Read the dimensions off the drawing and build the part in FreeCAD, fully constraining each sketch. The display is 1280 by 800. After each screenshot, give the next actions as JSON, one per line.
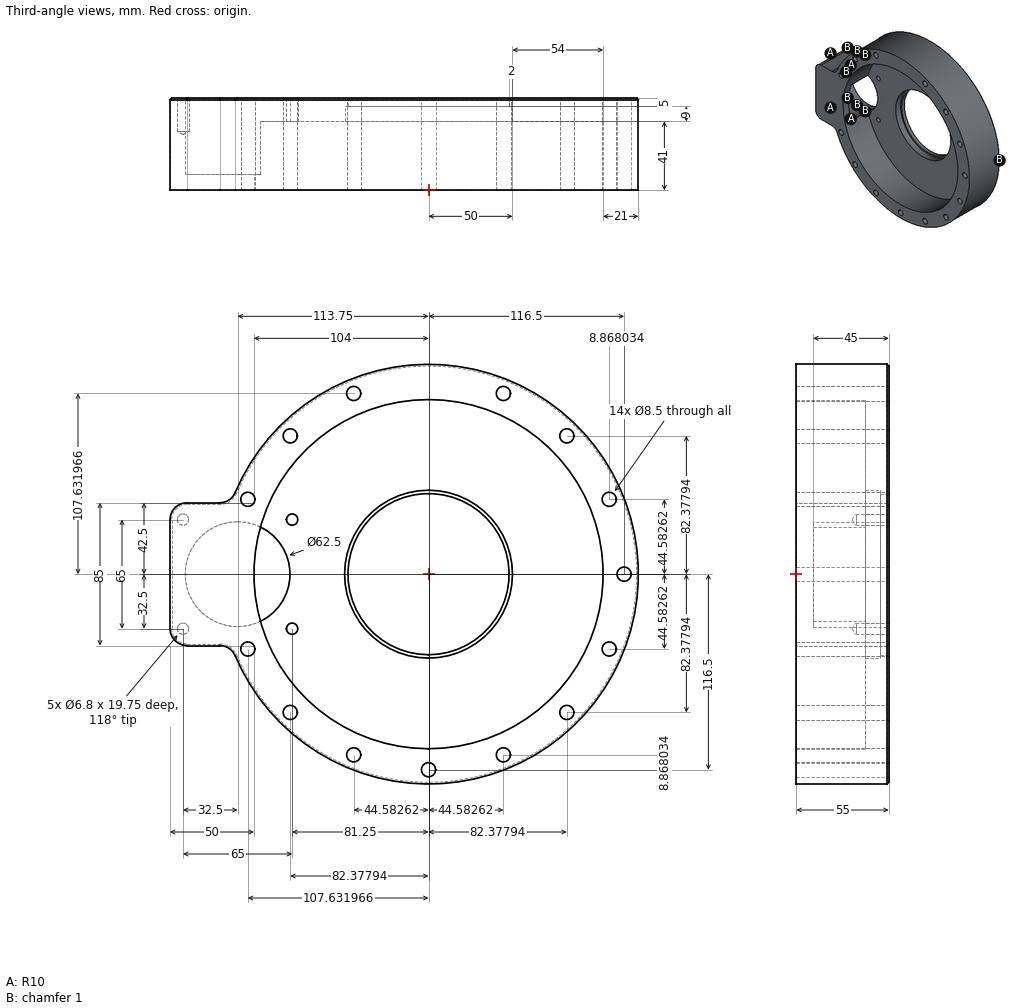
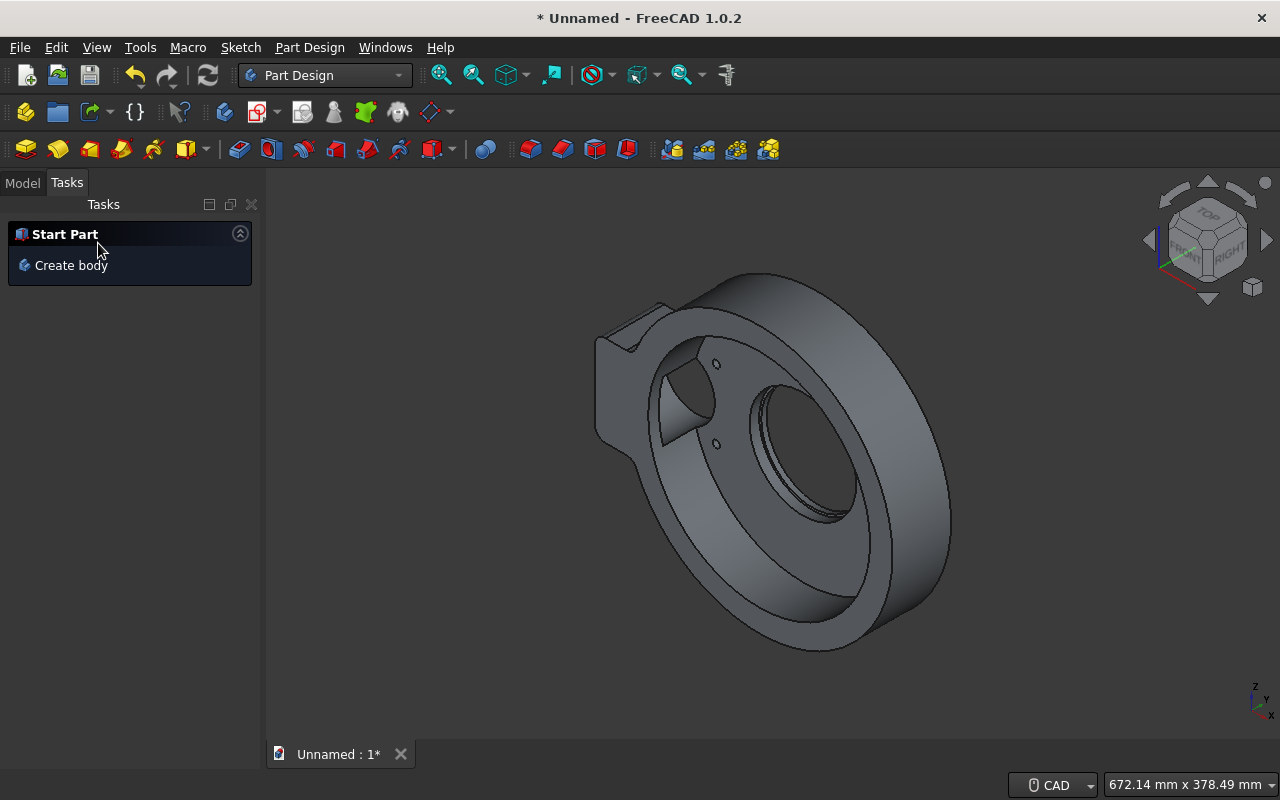
{"action": "left_click", "coordinate": [616, 396]}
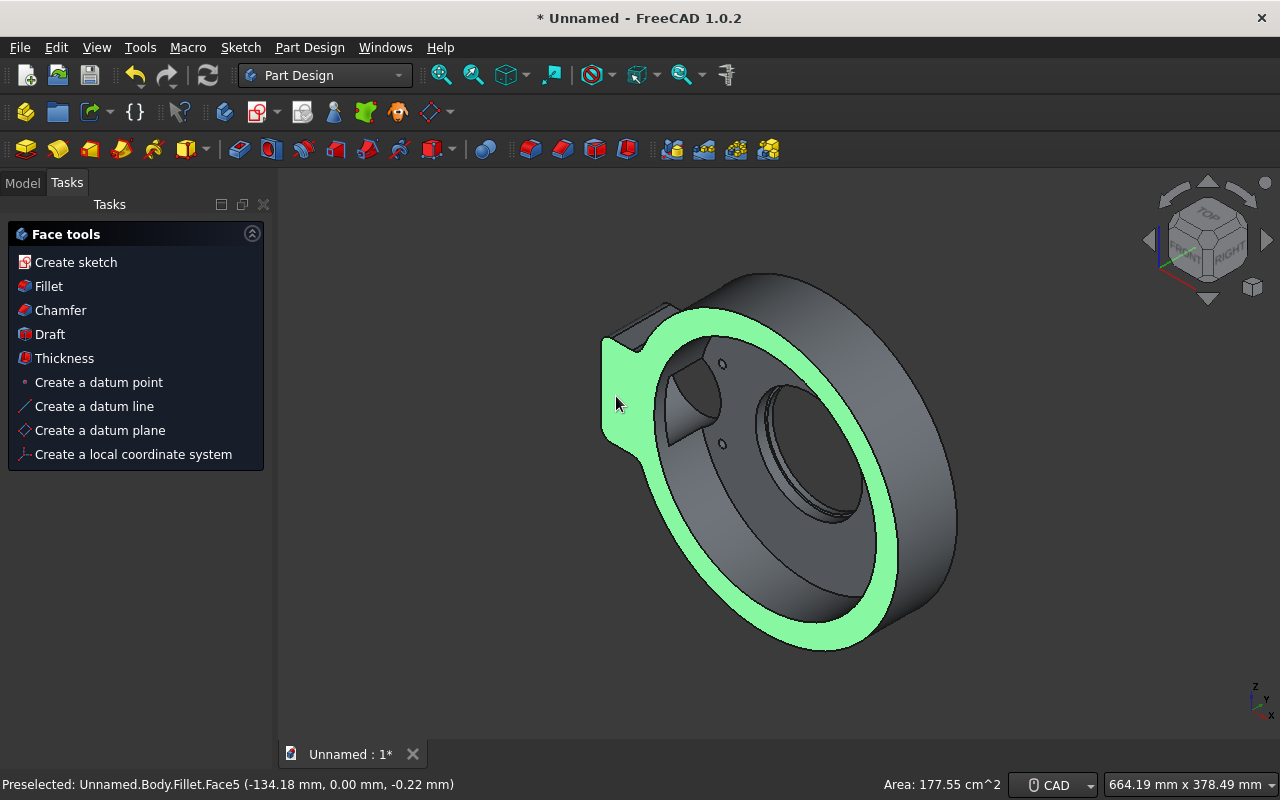
{"action": "left_click", "coordinate": [258, 112]}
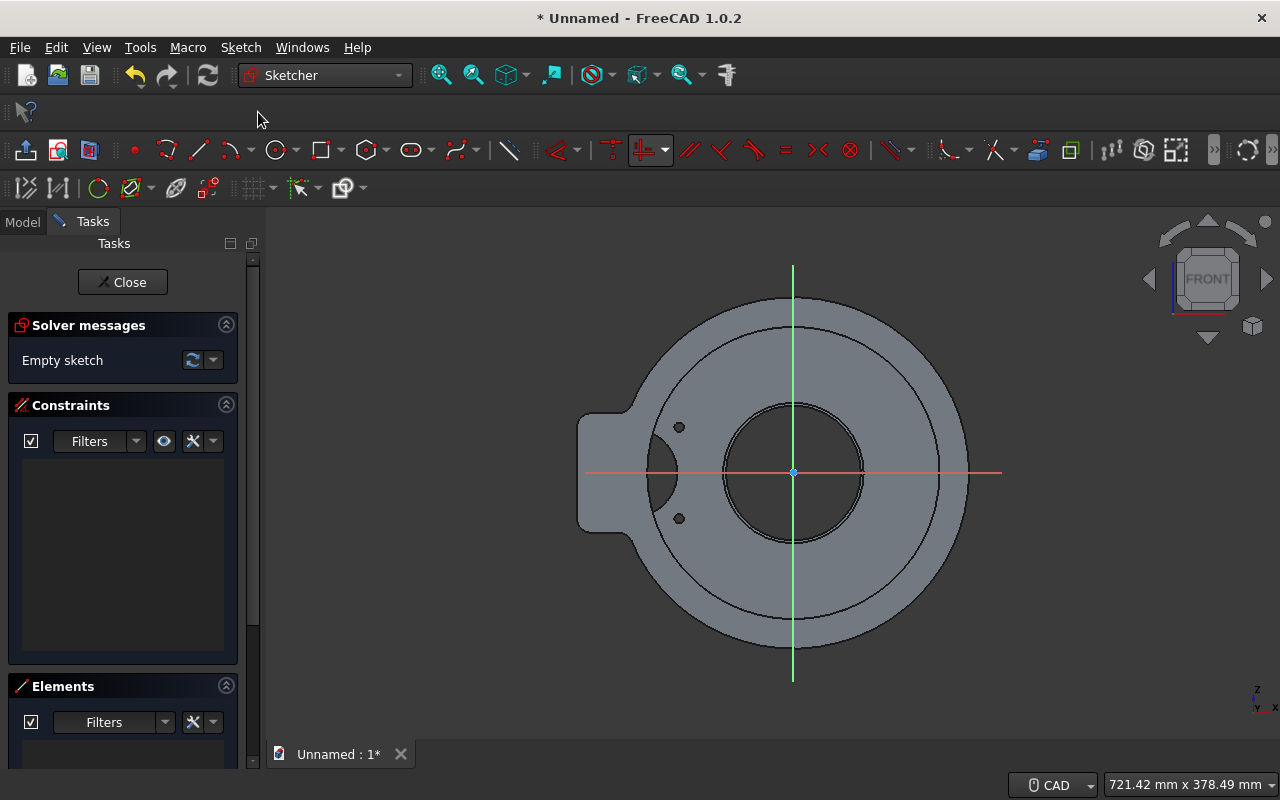
{"action": "key", "text": "g c"}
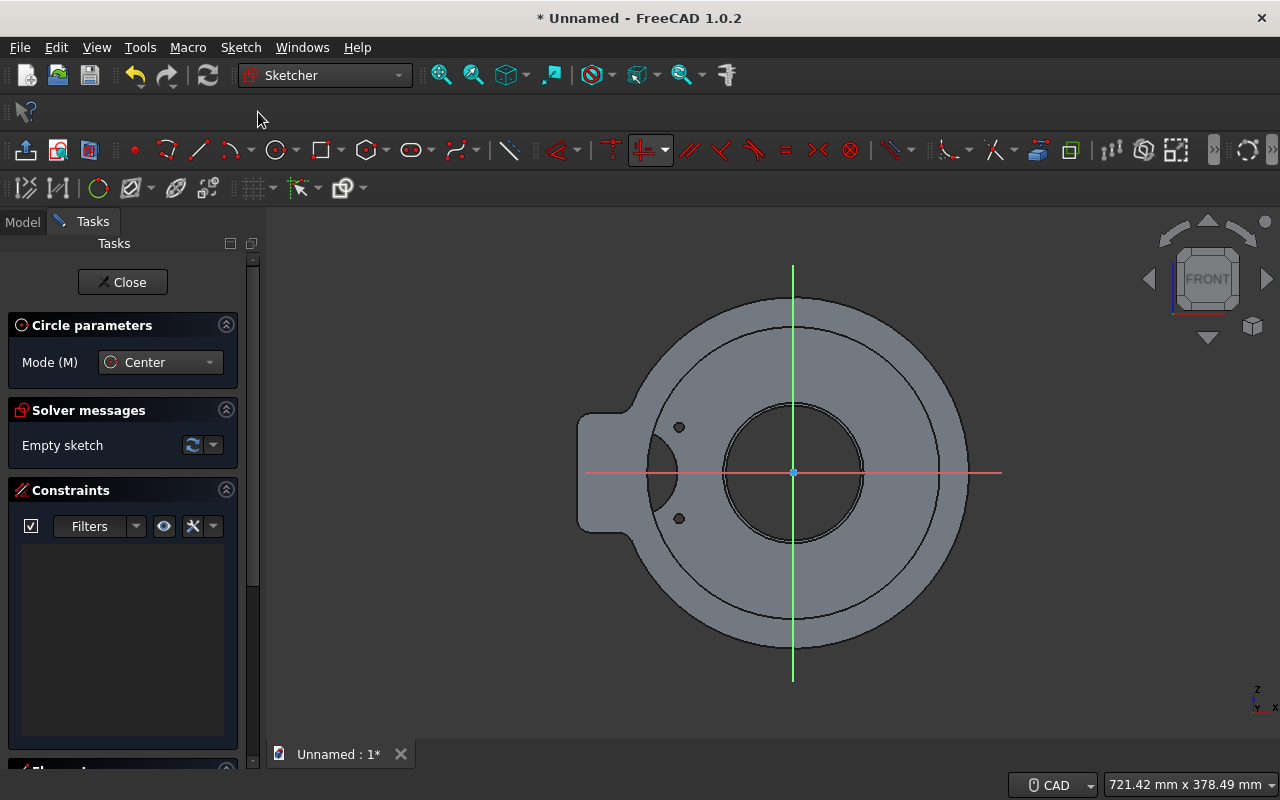
{"action": "scroll", "coordinate": [945, 410], "scroll_direction": "up", "scroll_amount": 7}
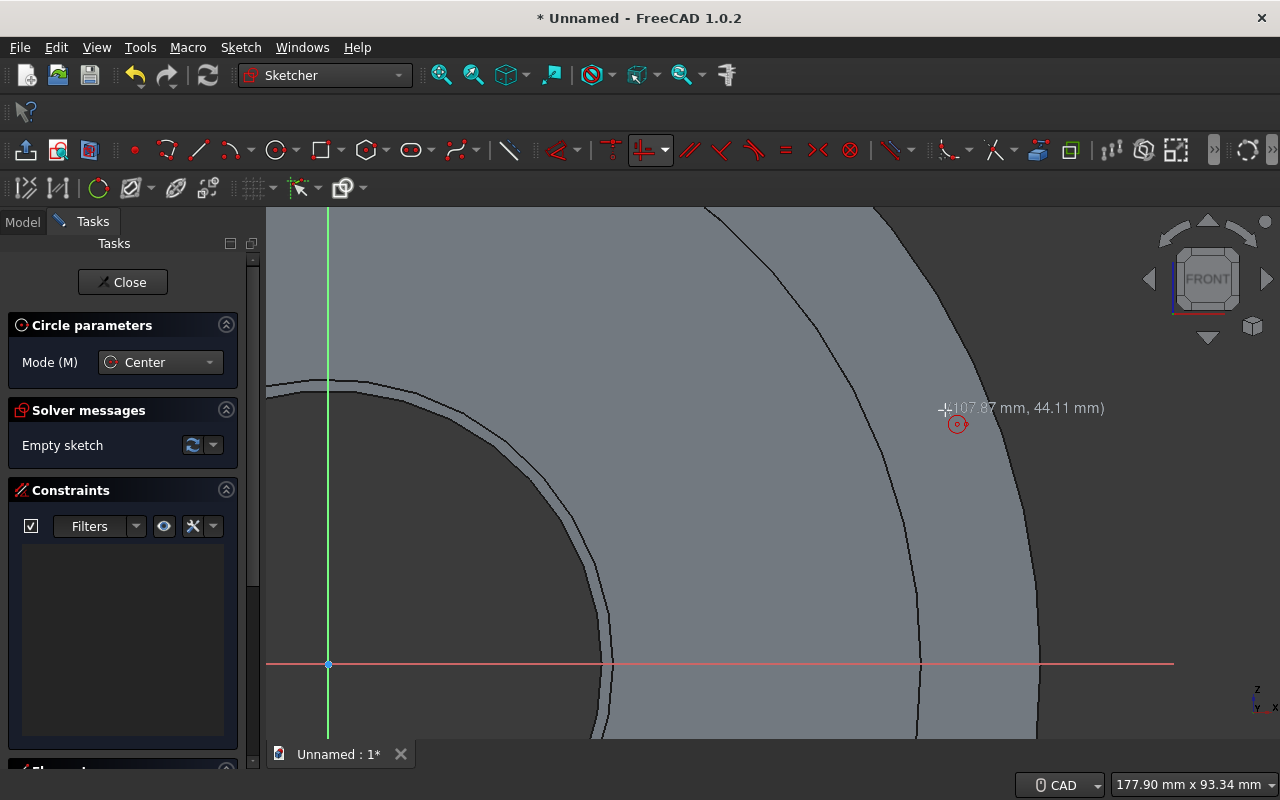
{"action": "scroll", "coordinate": [819, 402], "scroll_direction": "down", "scroll_amount": 7}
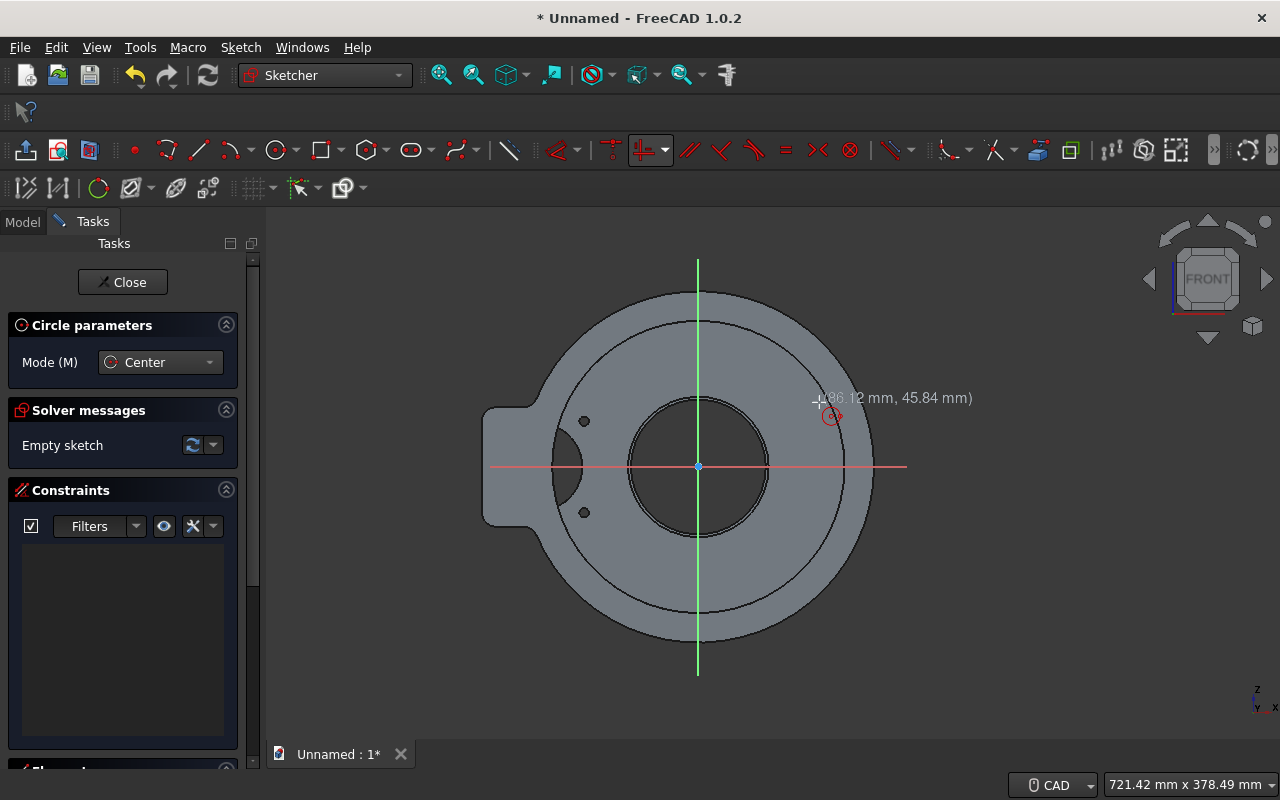
{"action": "left_click", "coordinate": [850, 404]}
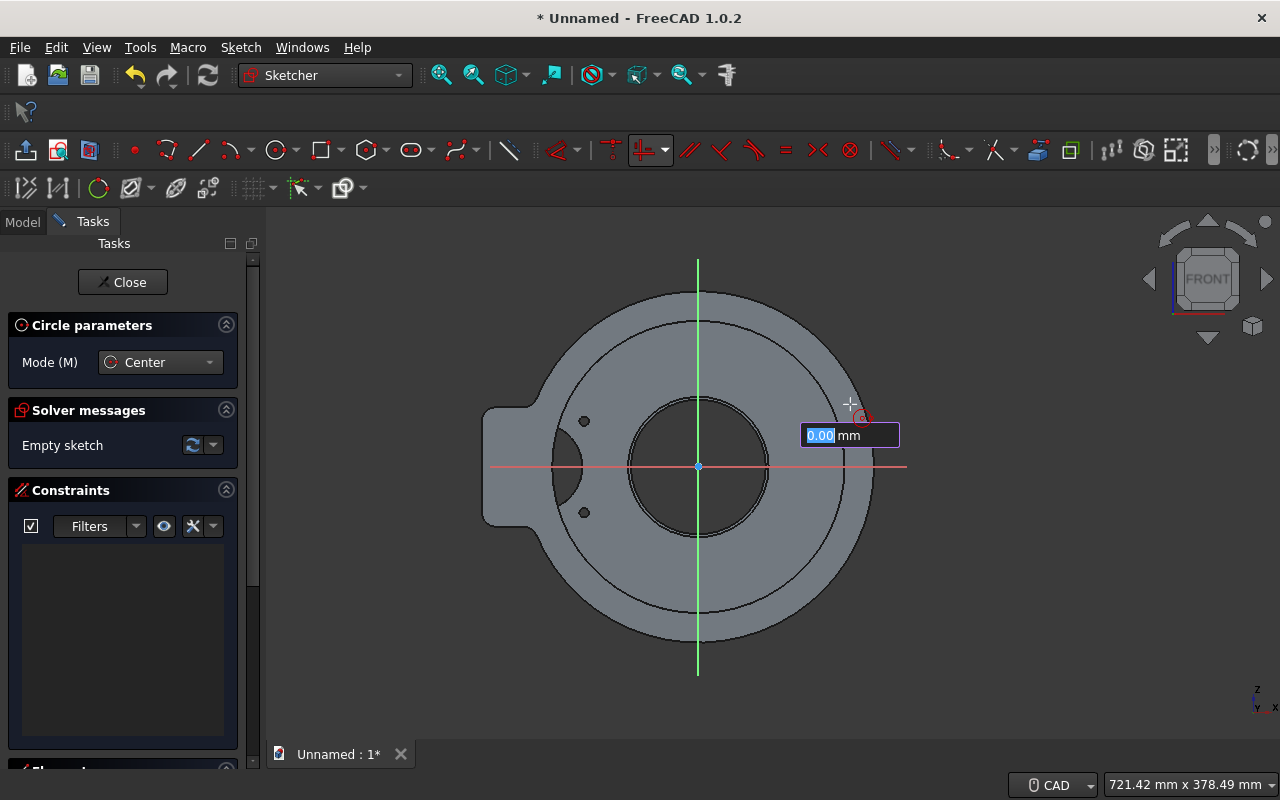
{"action": "scroll", "coordinate": [854, 400], "scroll_direction": "up", "scroll_amount": 5}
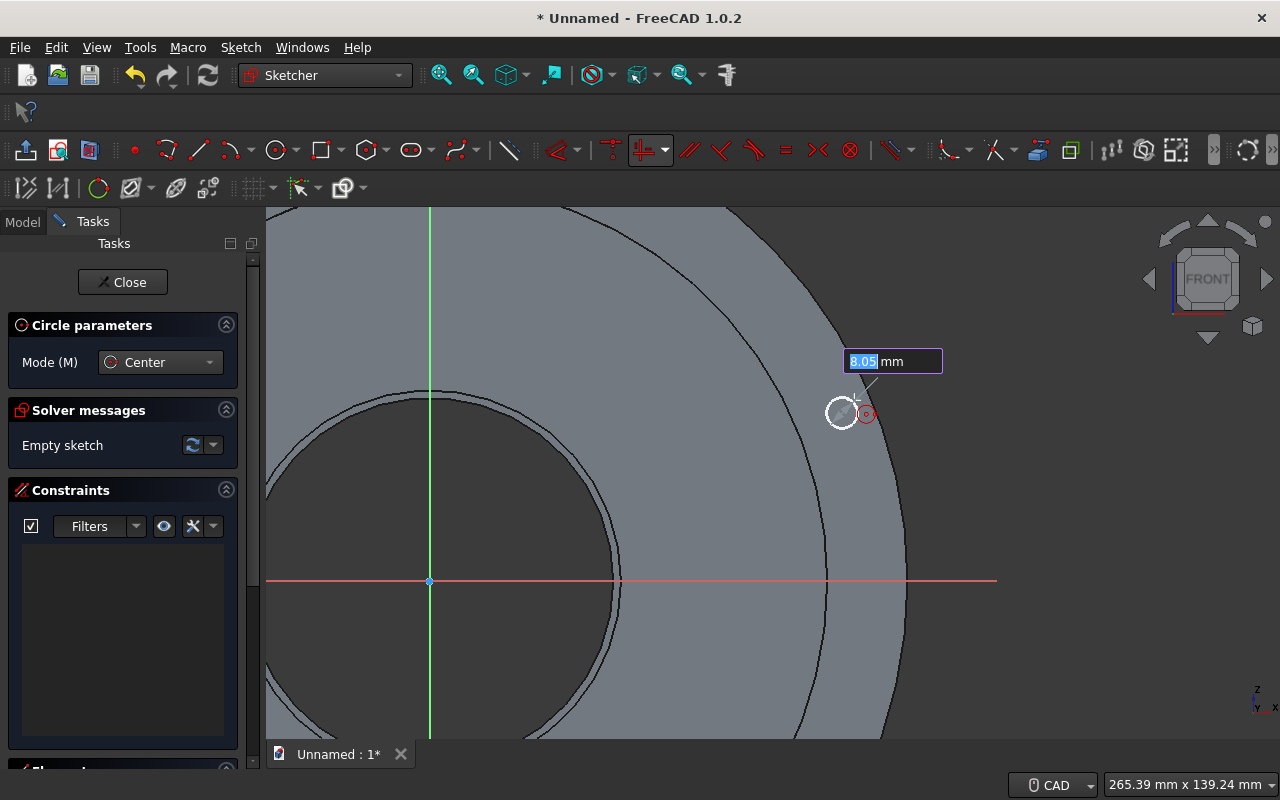
{"action": "left_click", "coordinate": [853, 400]}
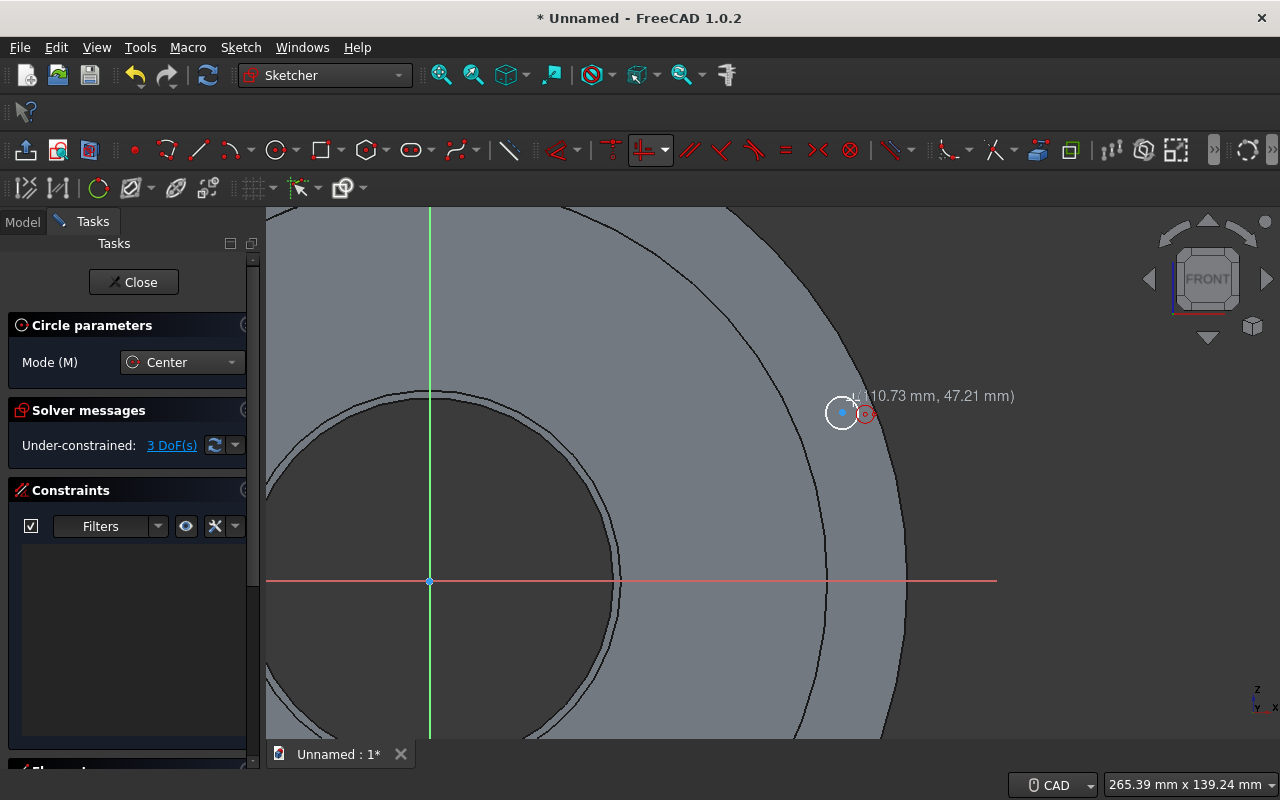
{"action": "scroll", "coordinate": [854, 400], "scroll_direction": "down", "scroll_amount": 5}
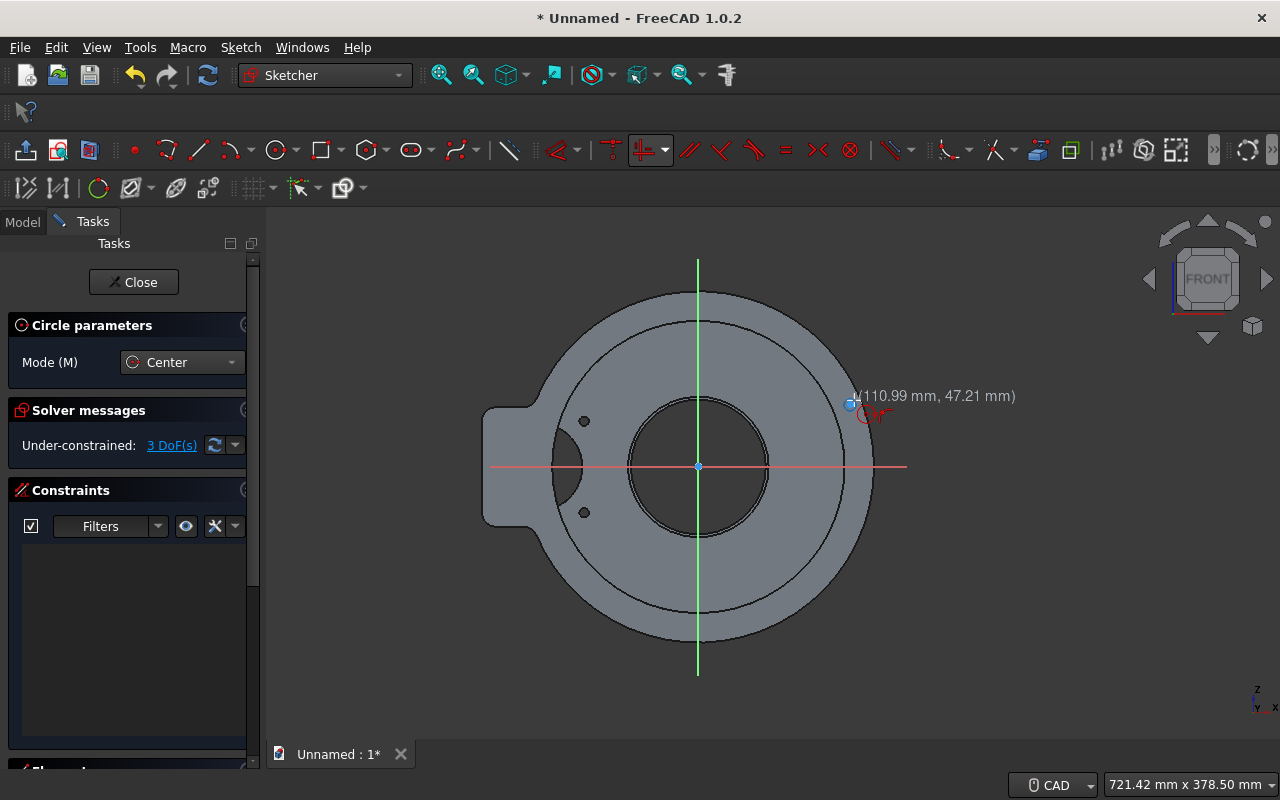
{"action": "scroll", "coordinate": [850, 530], "scroll_direction": "up", "scroll_amount": 7}